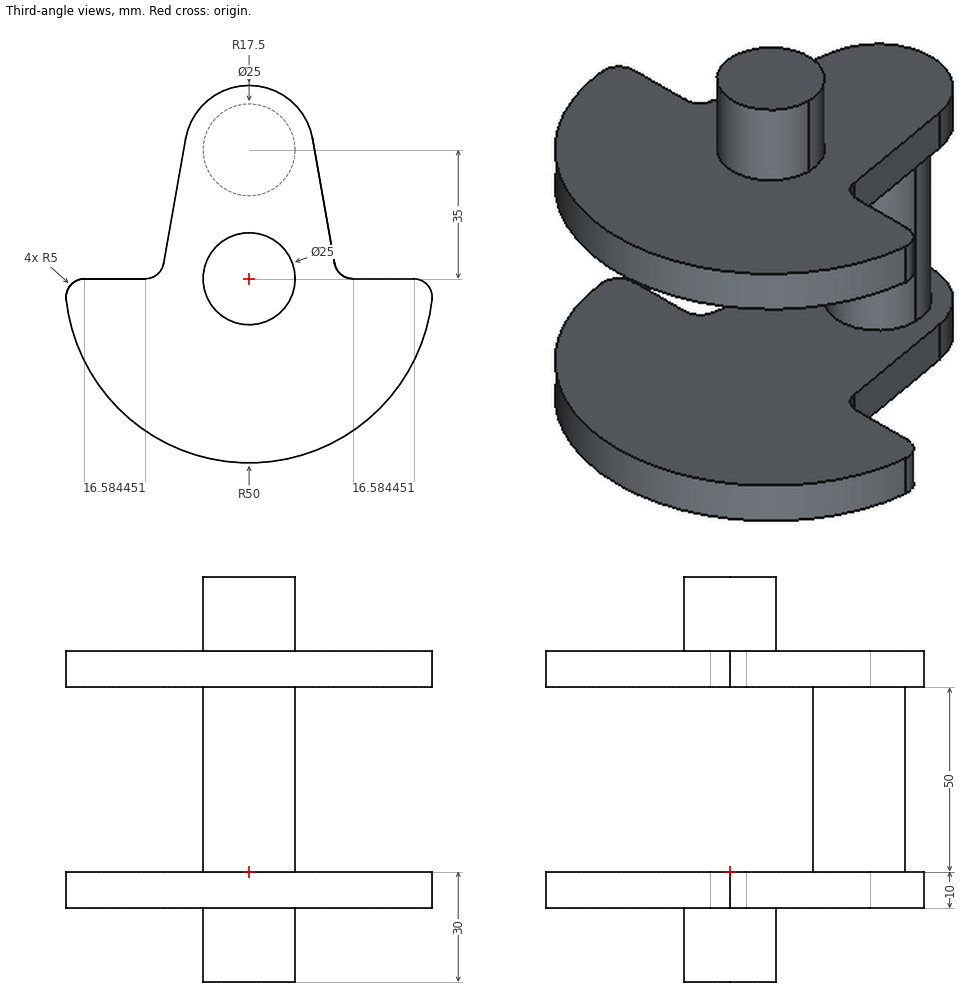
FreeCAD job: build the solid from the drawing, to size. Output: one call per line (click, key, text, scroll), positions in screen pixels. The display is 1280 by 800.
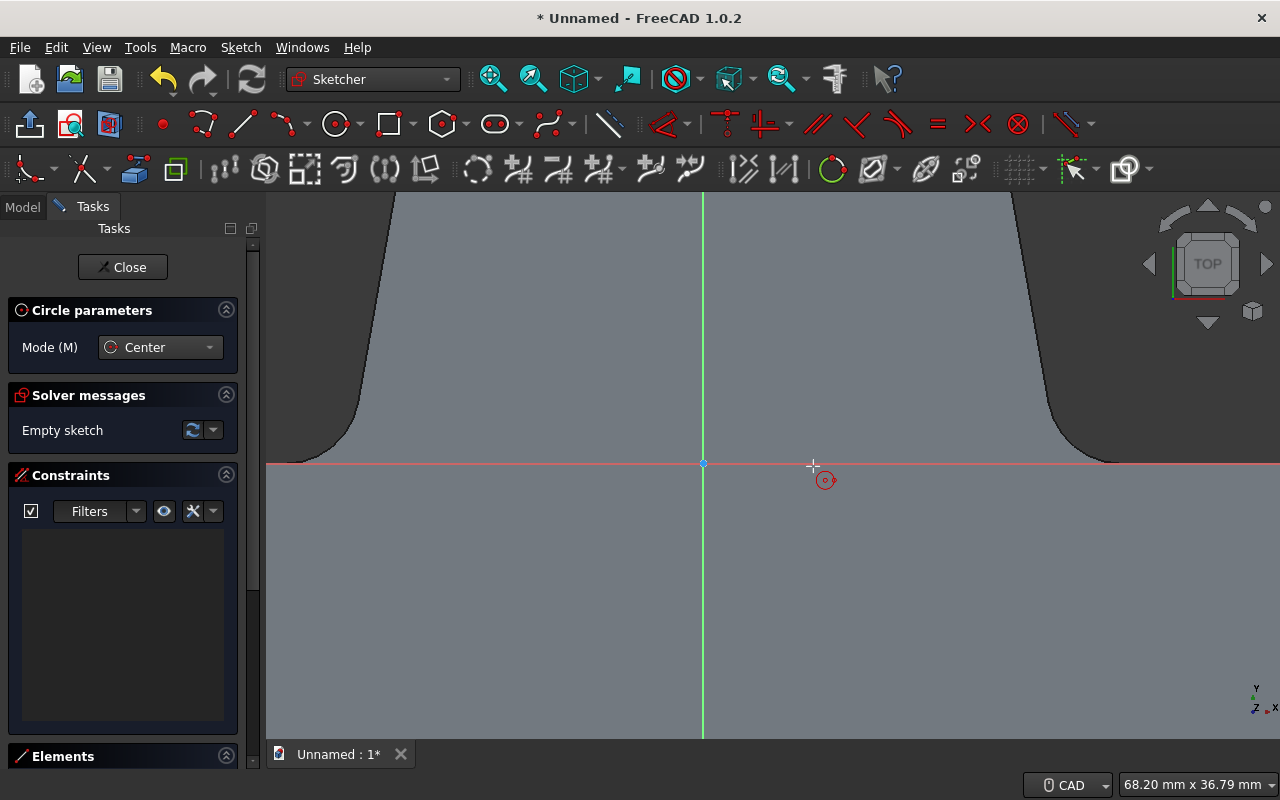
click(703, 464)
click(835, 332)
key(Escape)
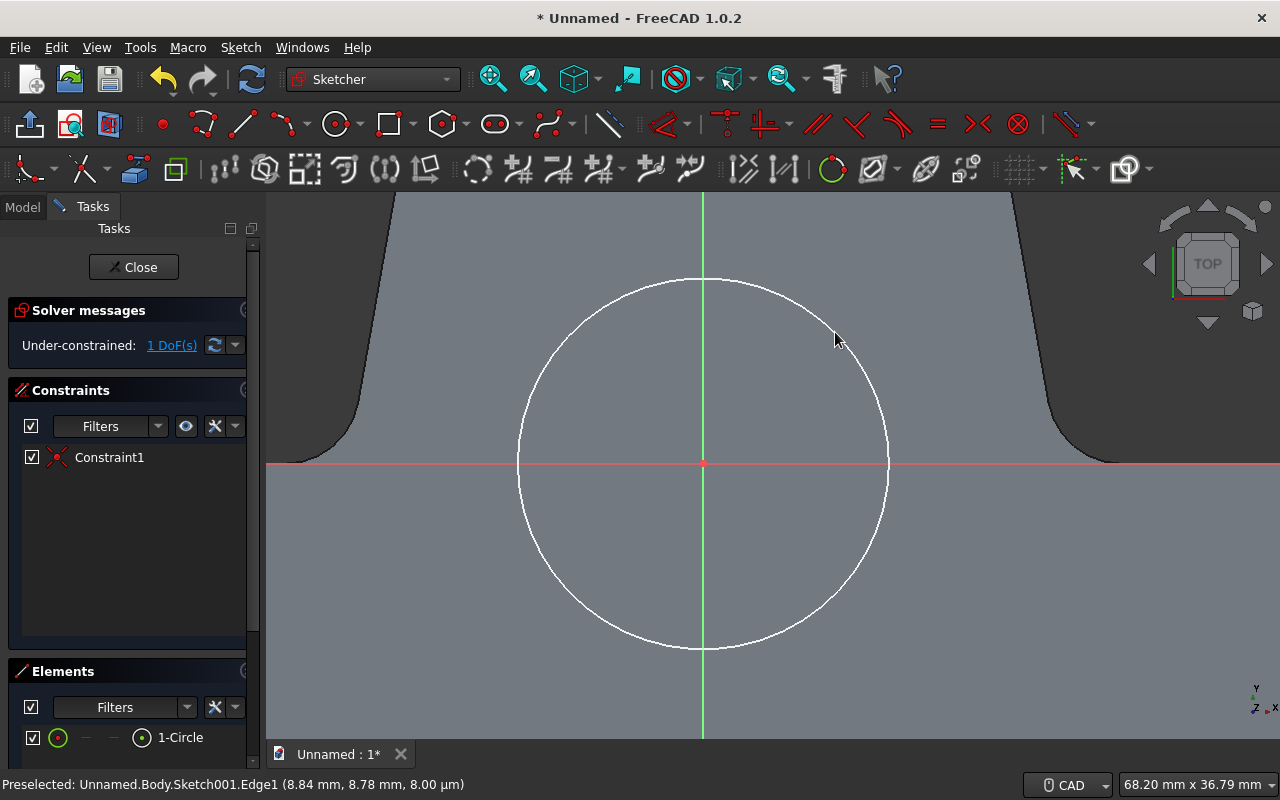
key(d)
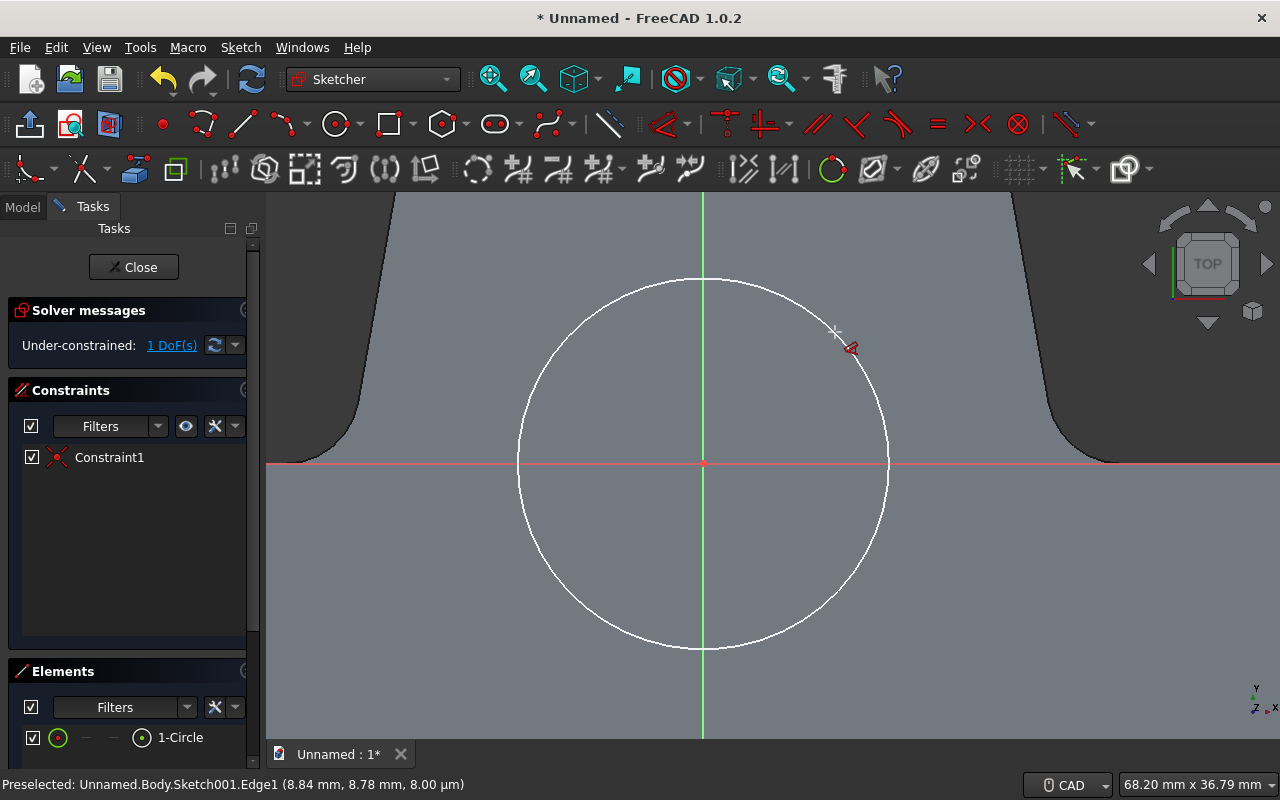
click(834, 332)
click(857, 309)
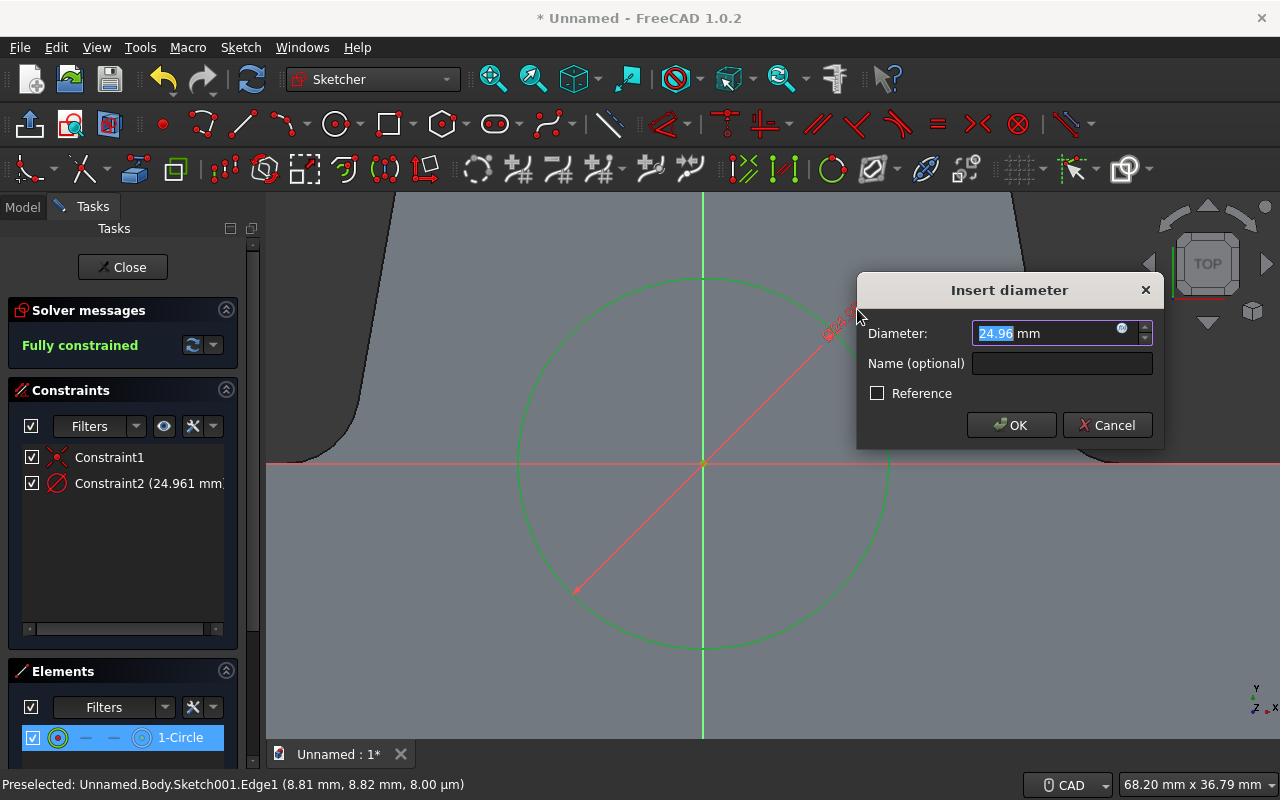
text(25)
key(Return)
key(Escape)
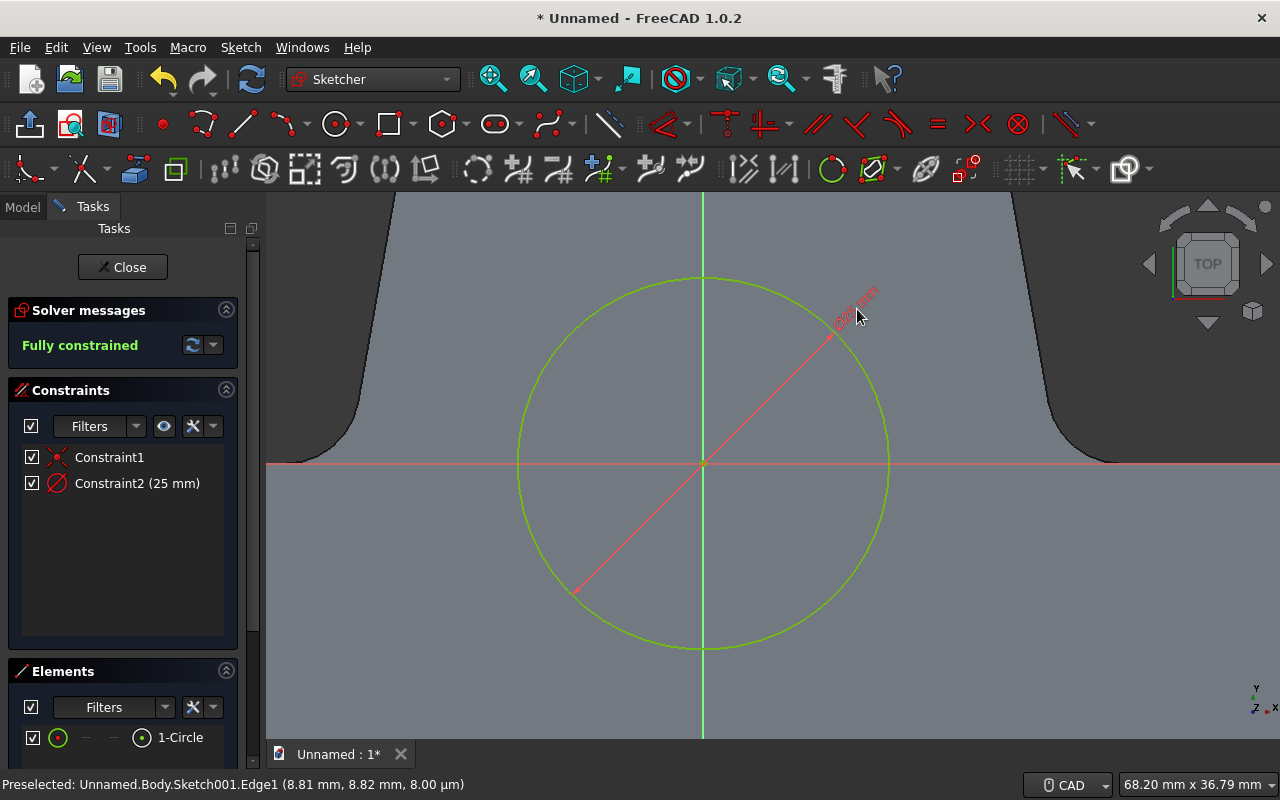
click(123, 267)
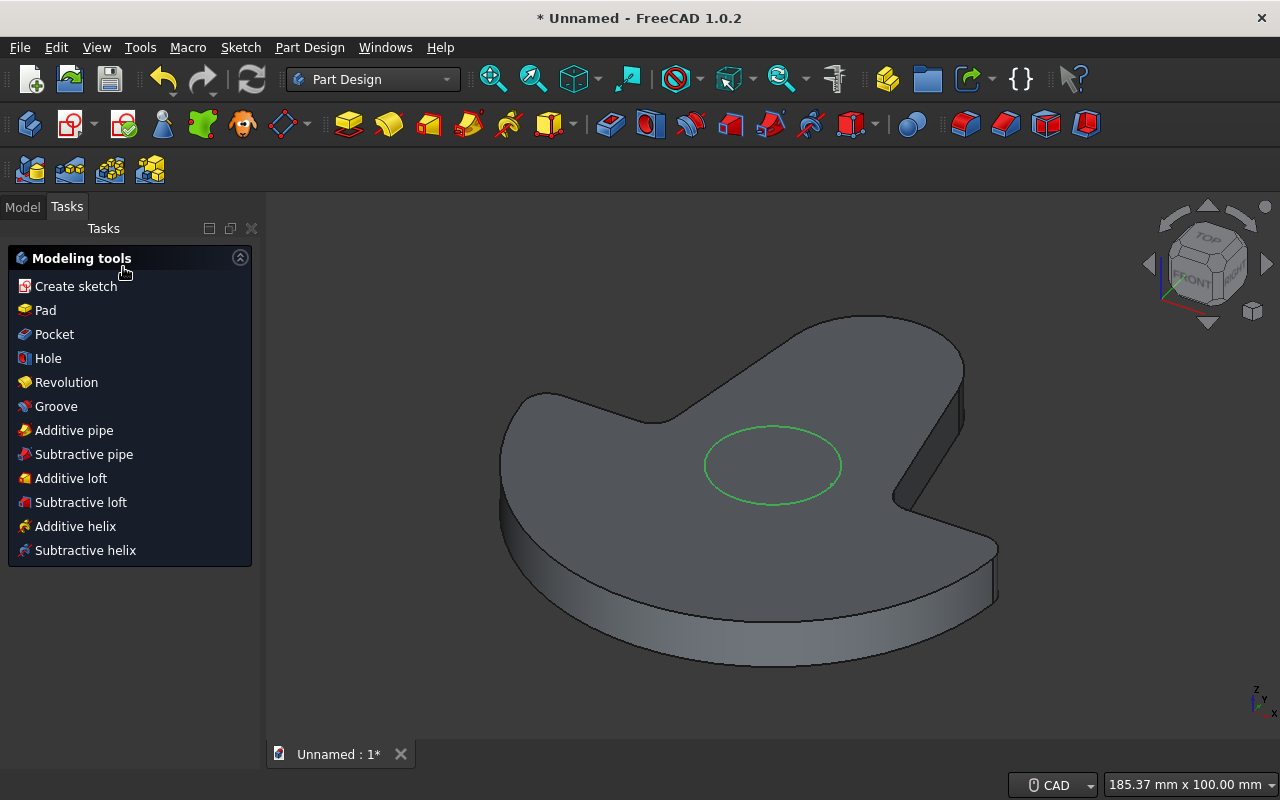
click(350, 124)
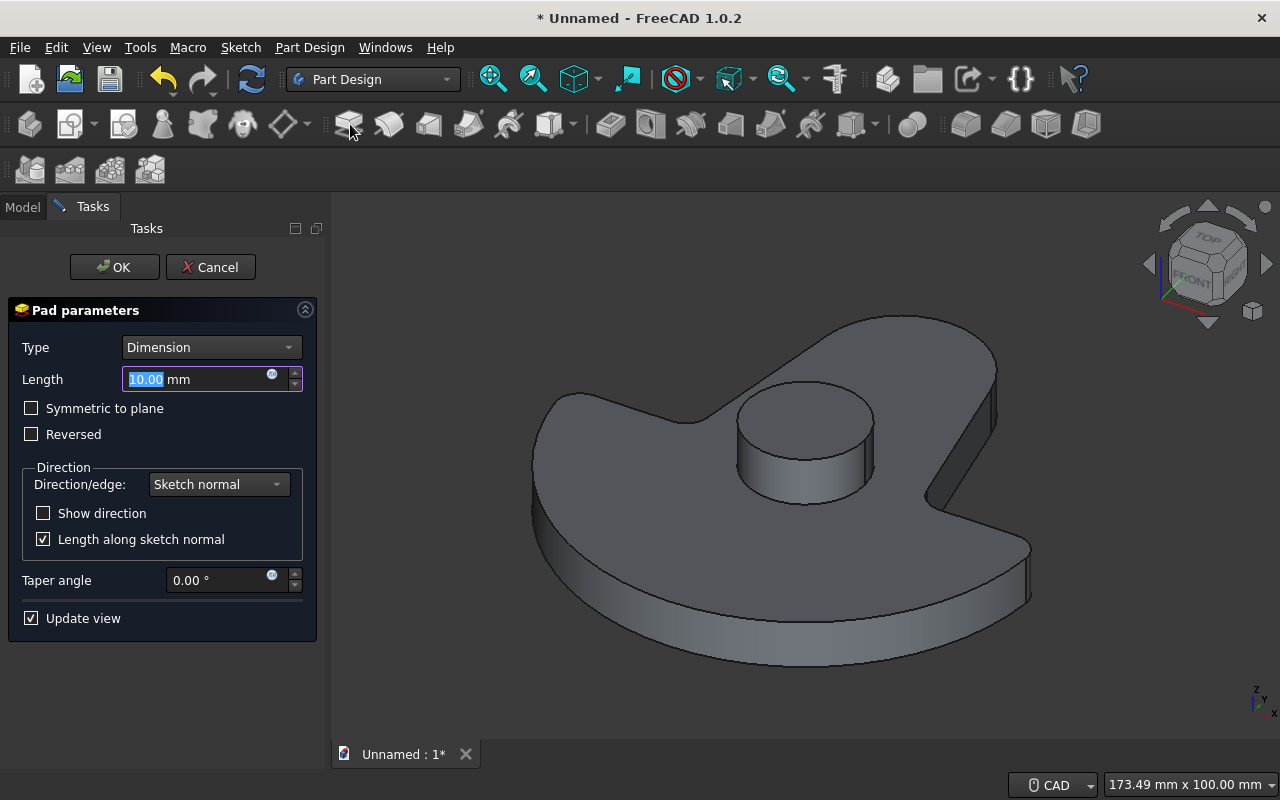
text(30)
key(Tab)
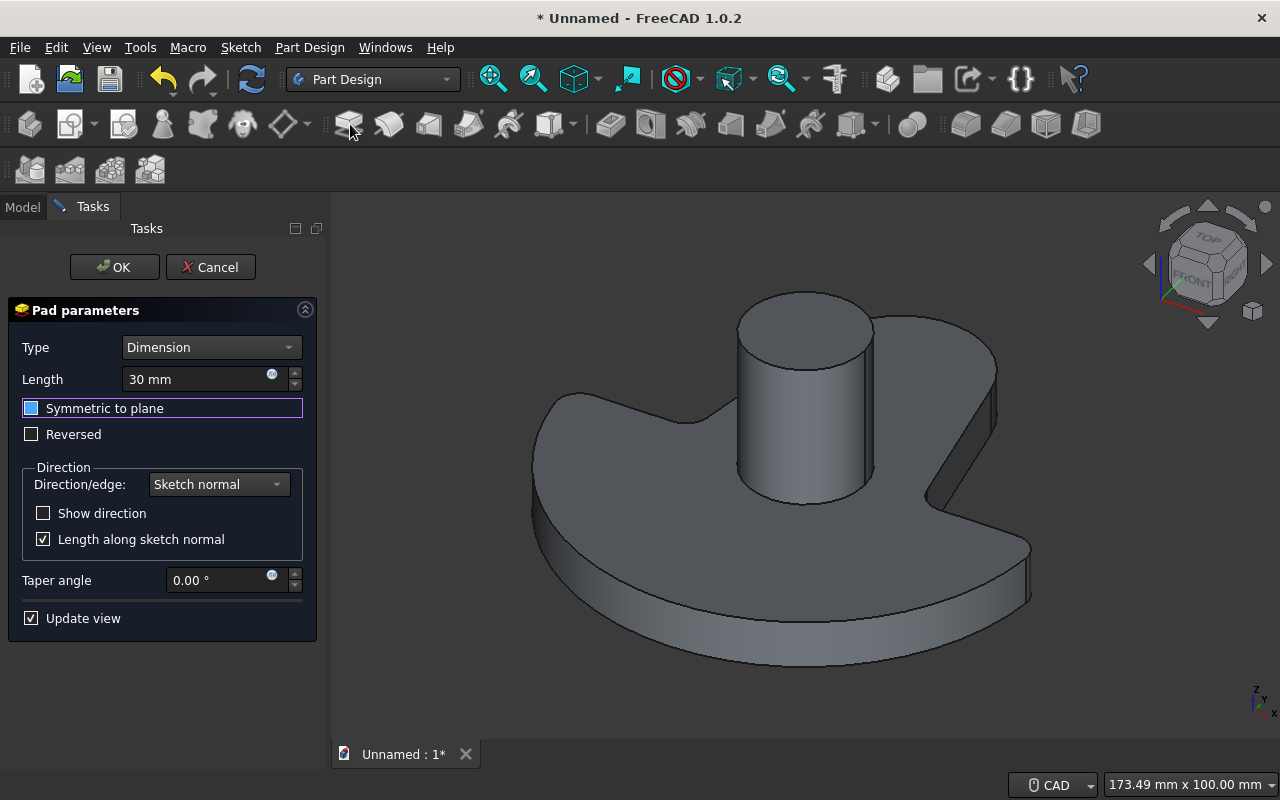
click(30, 434)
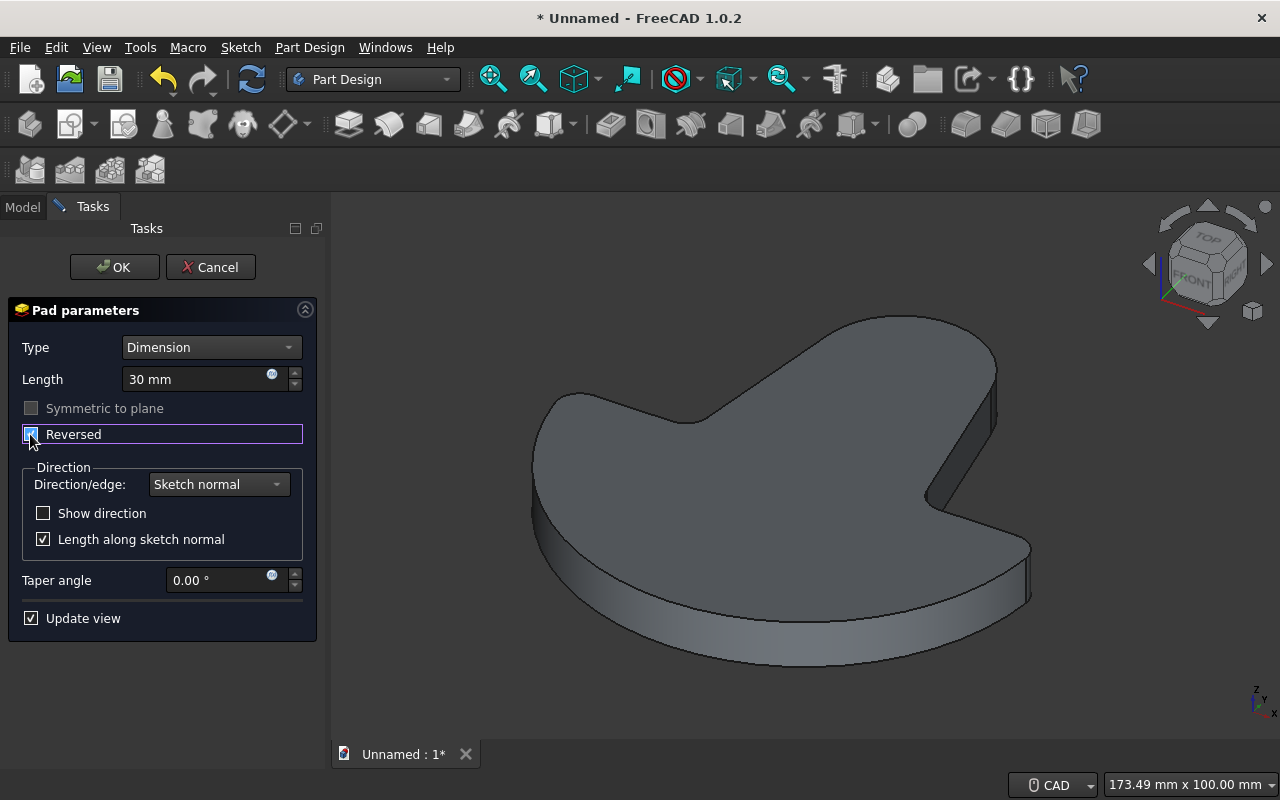
click(115, 267)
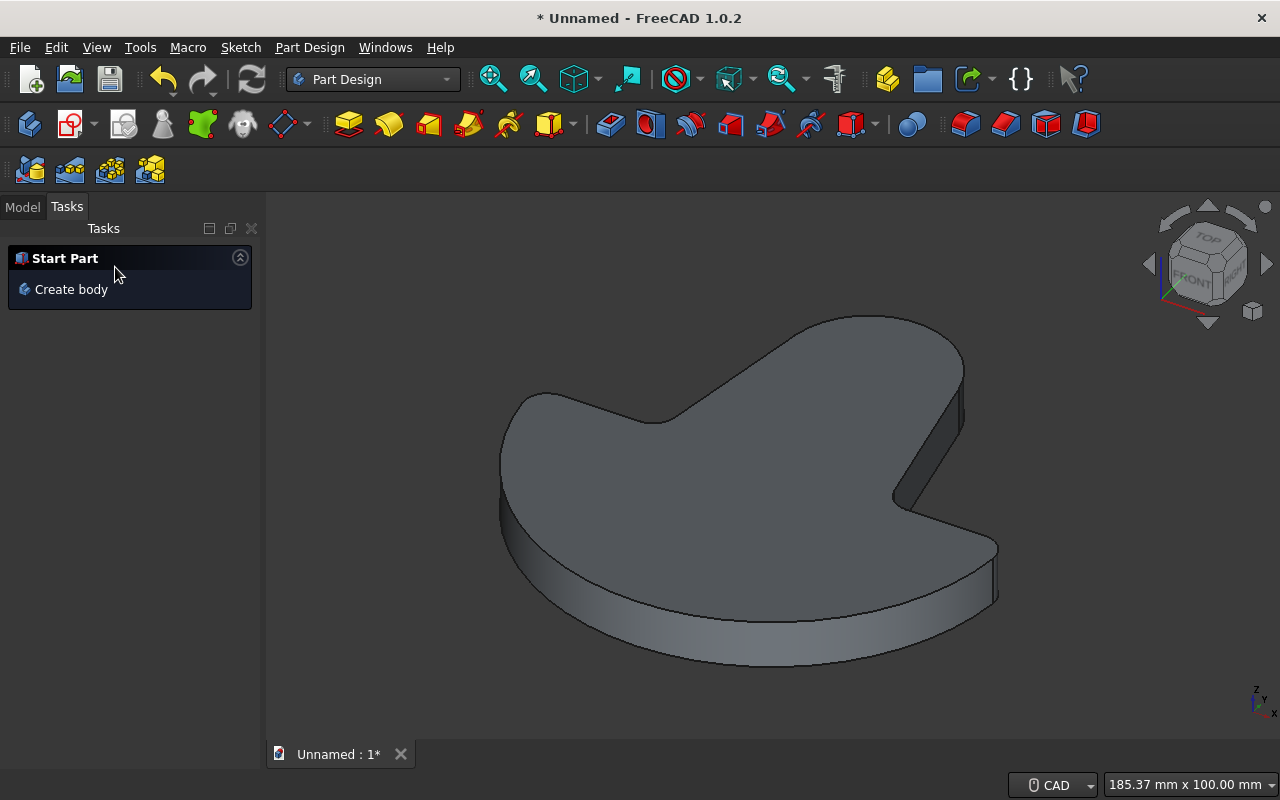
key(v)
key(f)